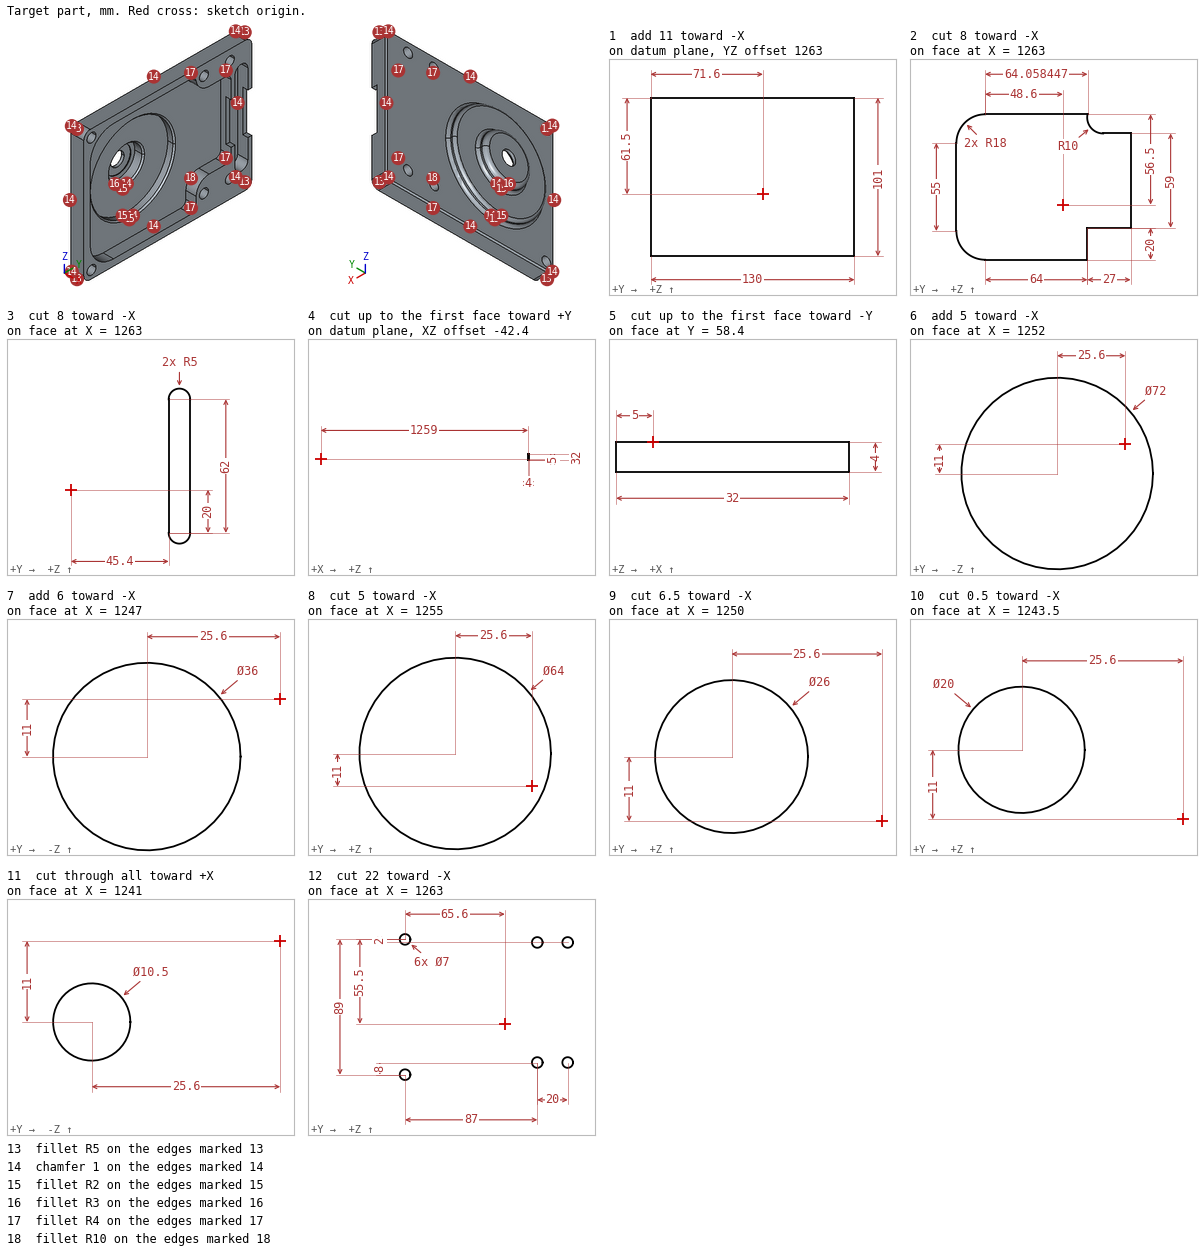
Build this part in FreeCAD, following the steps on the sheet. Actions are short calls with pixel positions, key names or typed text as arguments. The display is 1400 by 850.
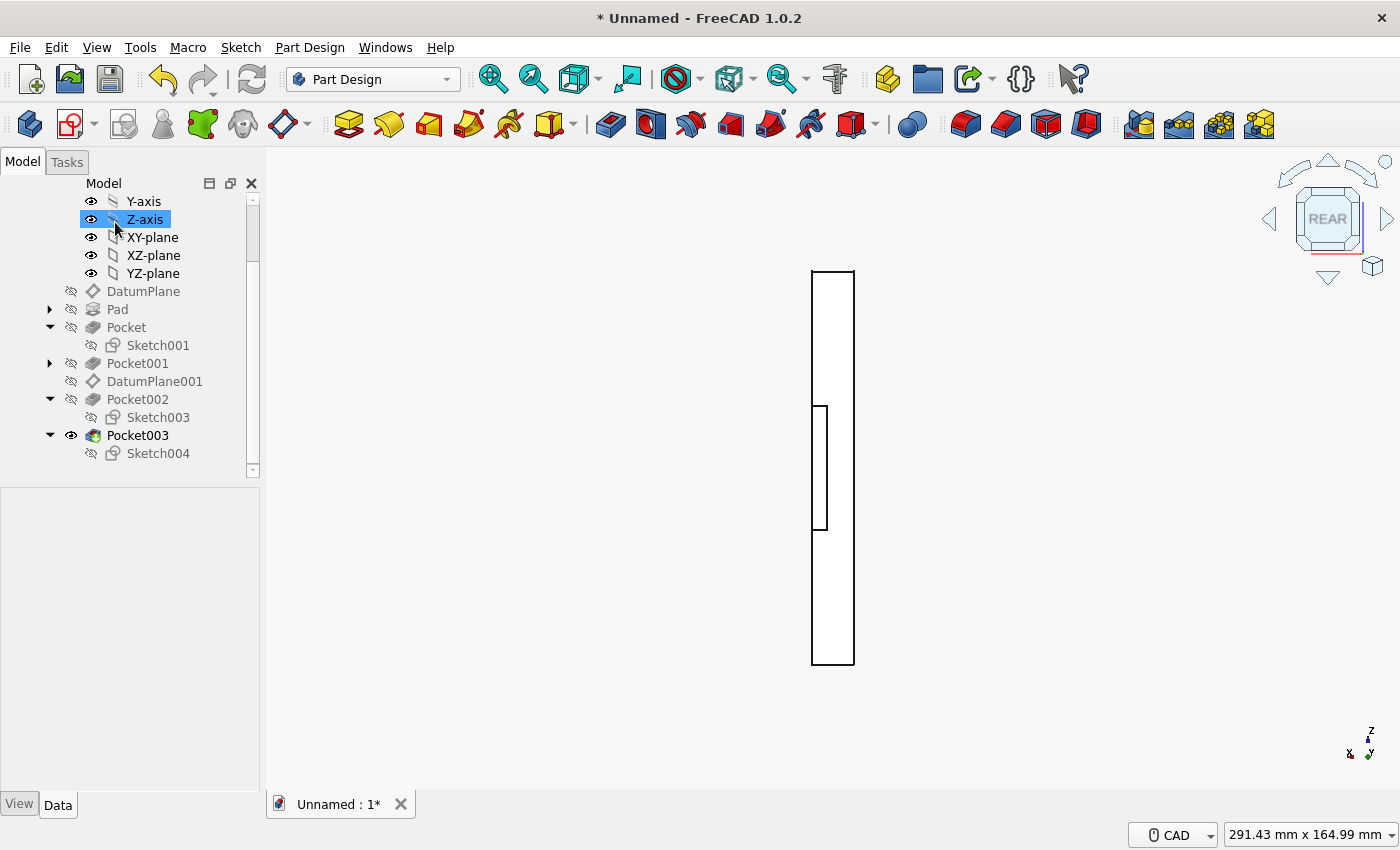
key(6)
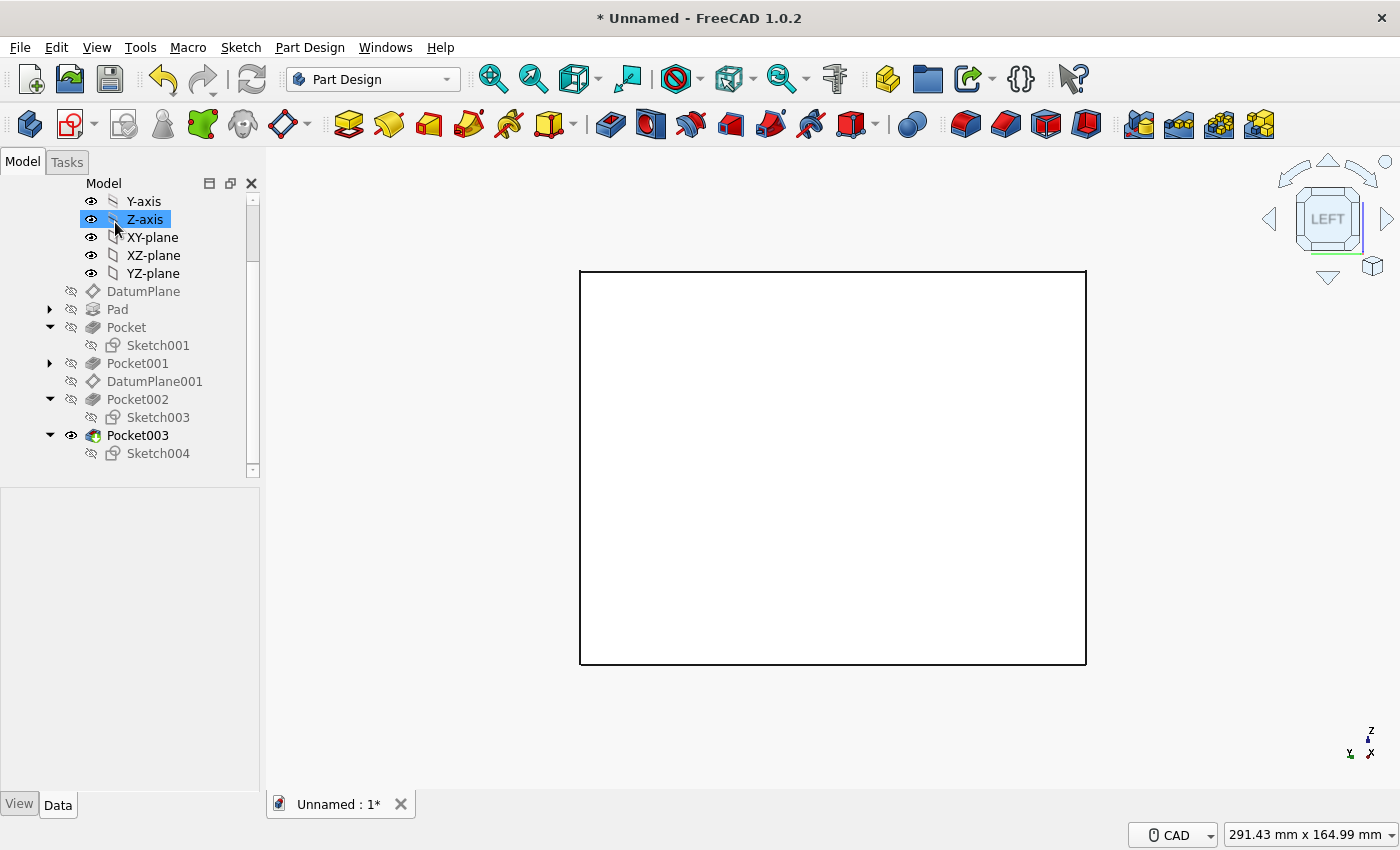
click(833, 467)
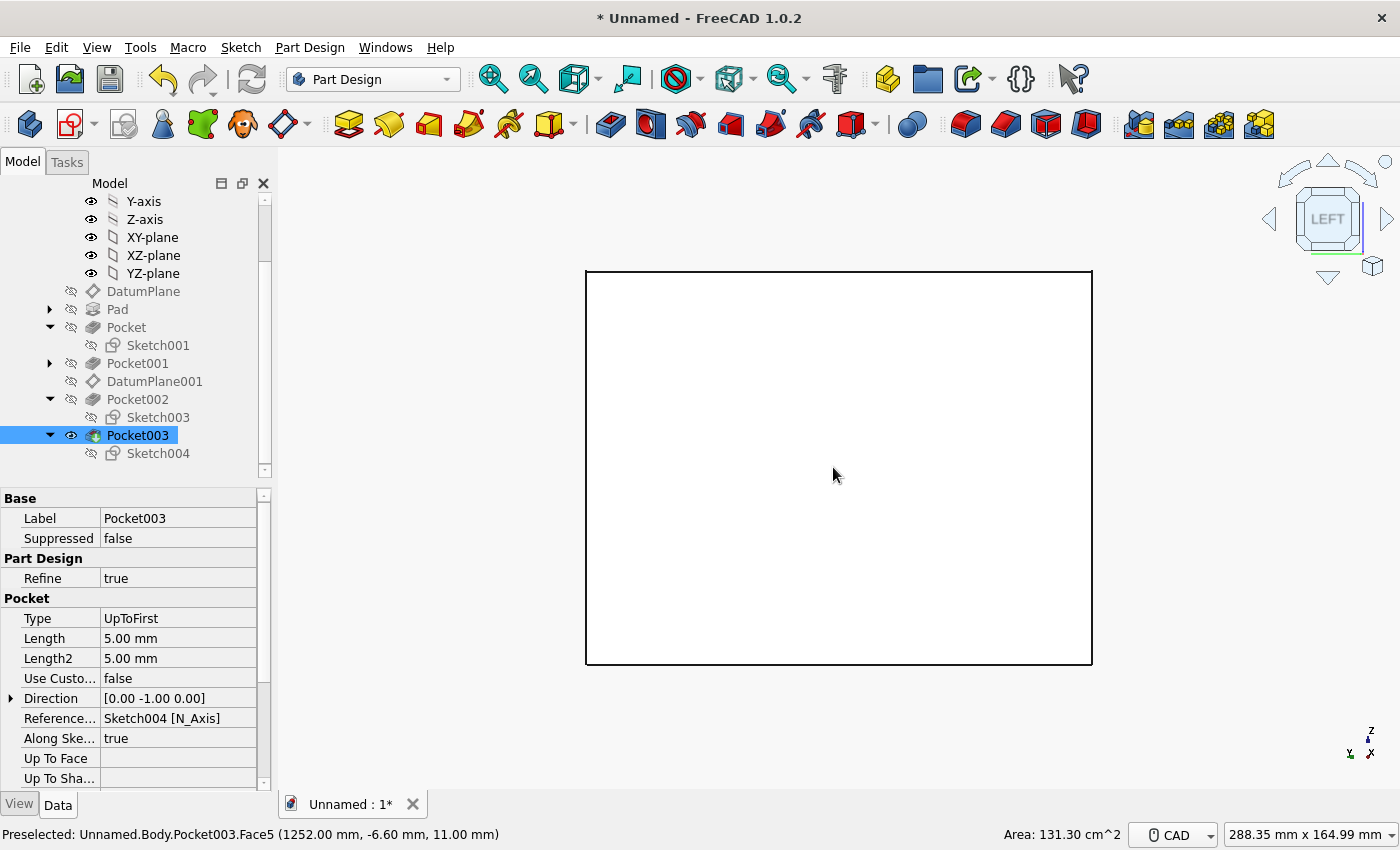
click(70, 124)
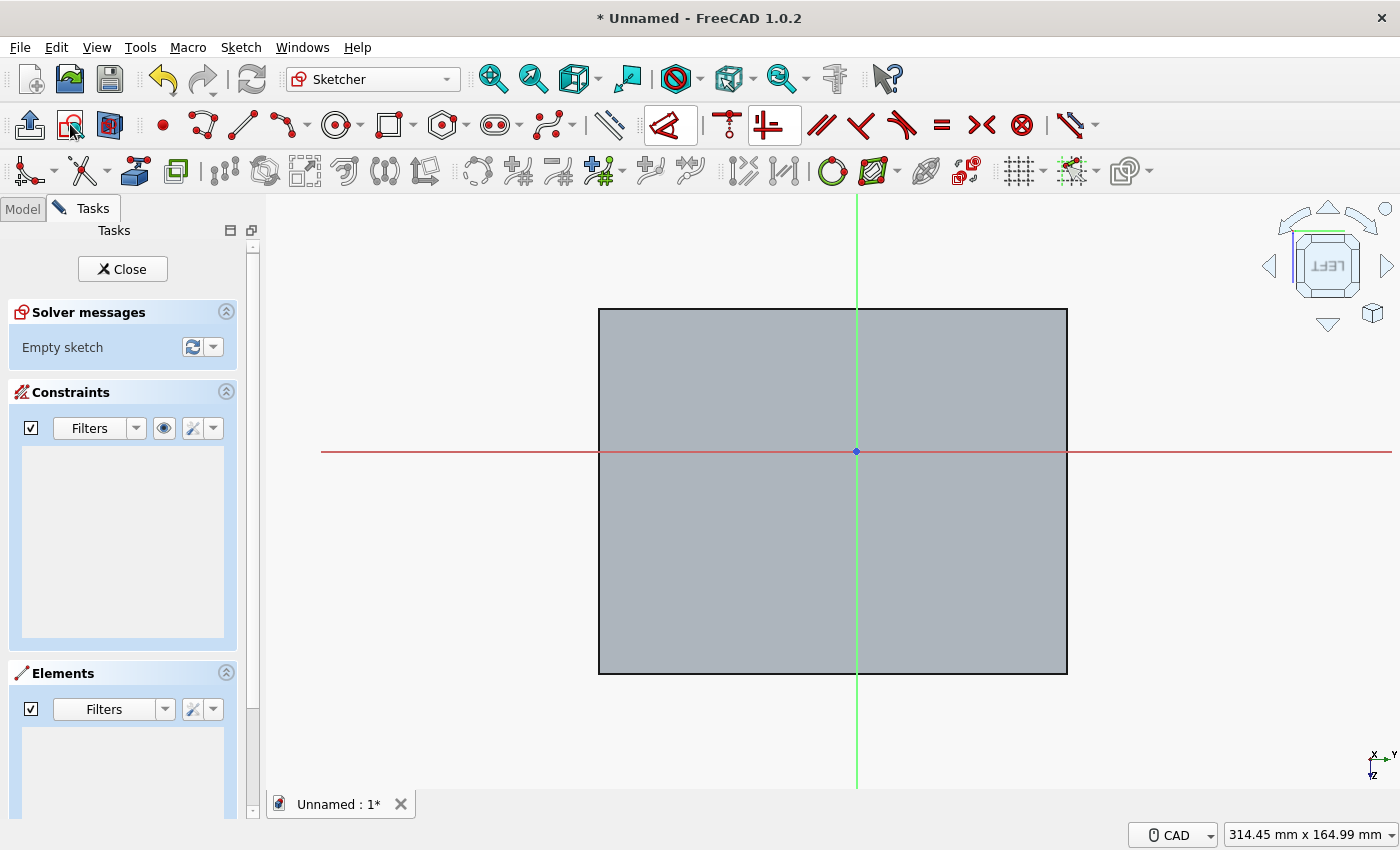
scroll(764, 491, up, 2)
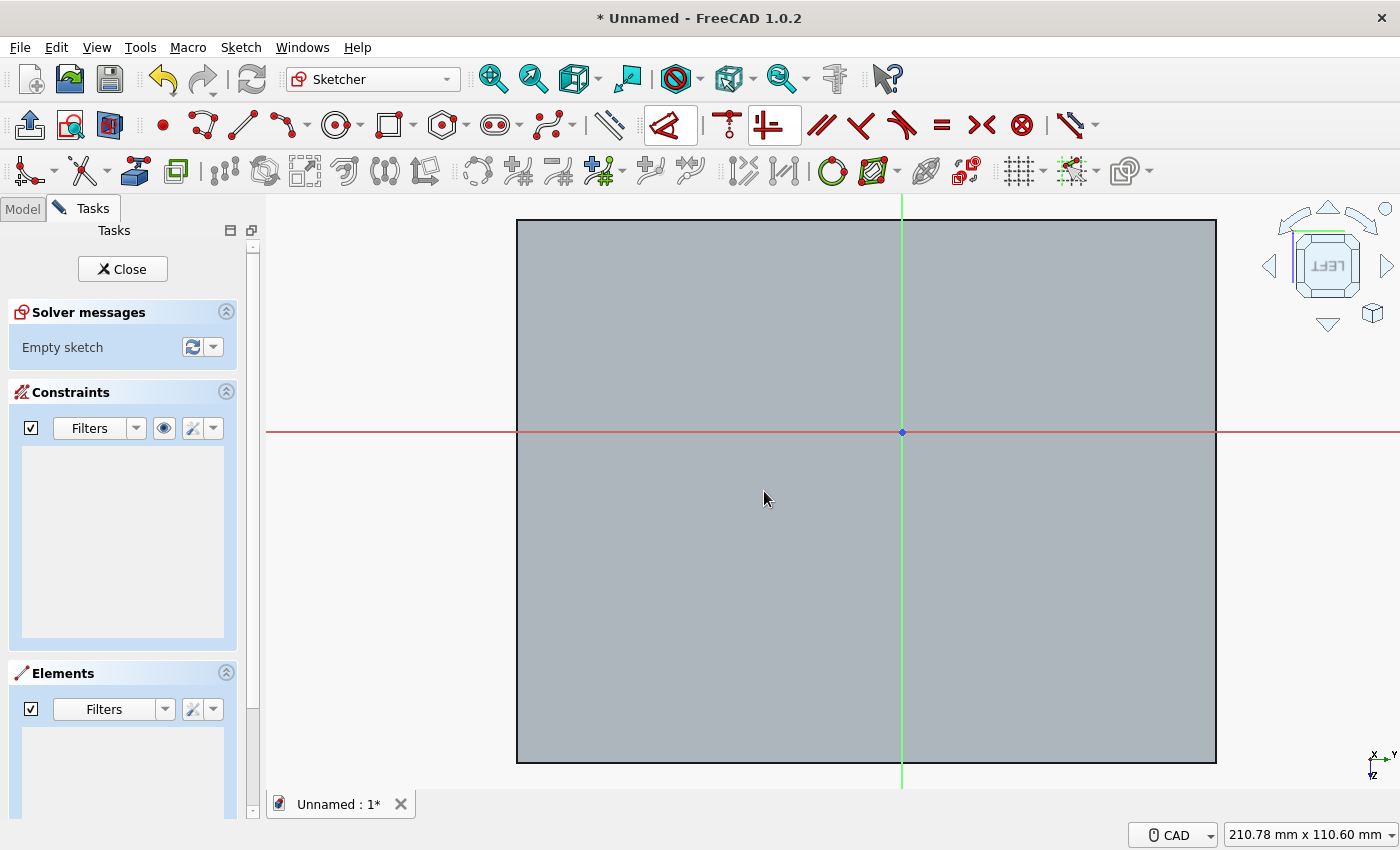
key(g)
key(c)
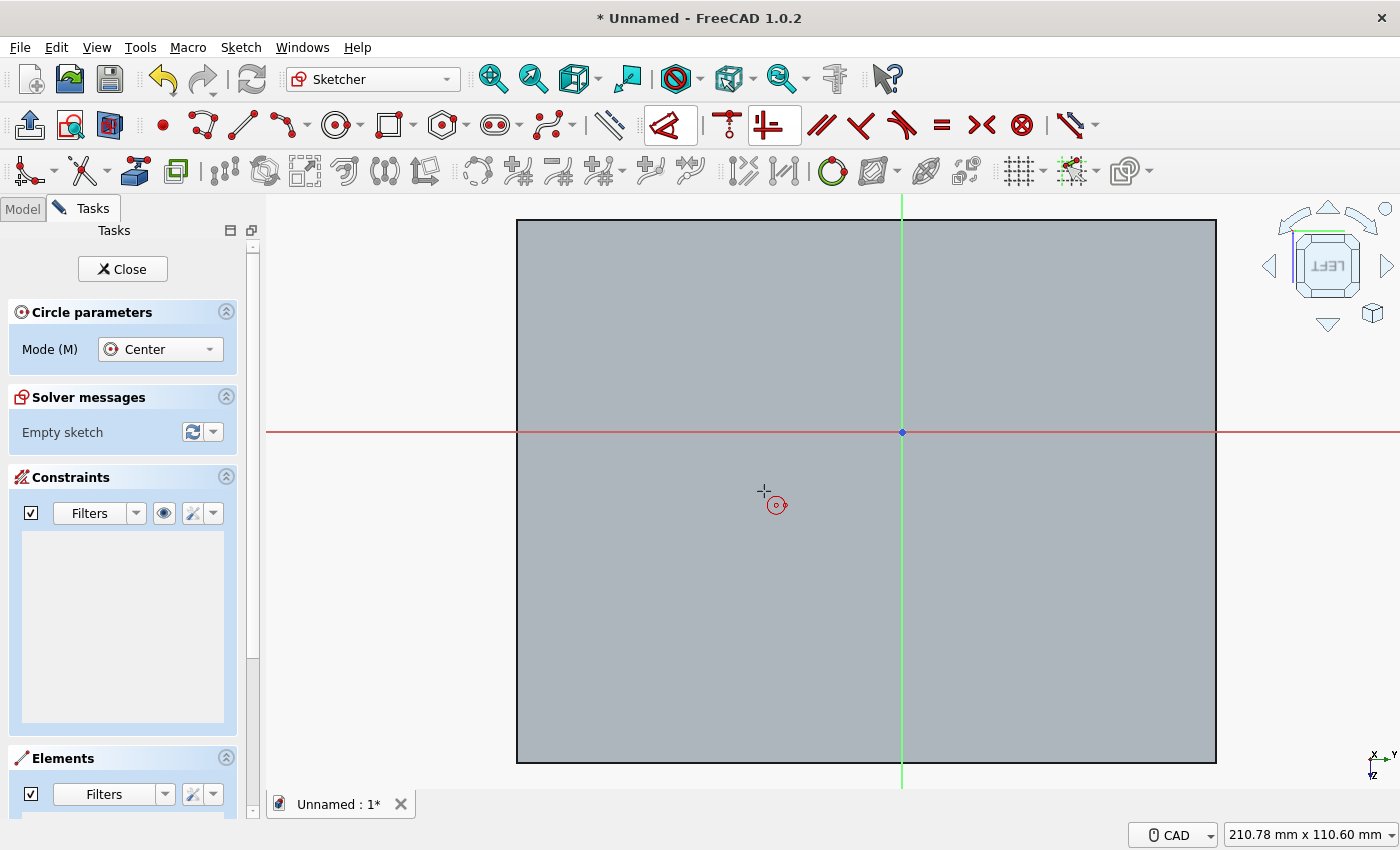
click(765, 491)
move(628, 355)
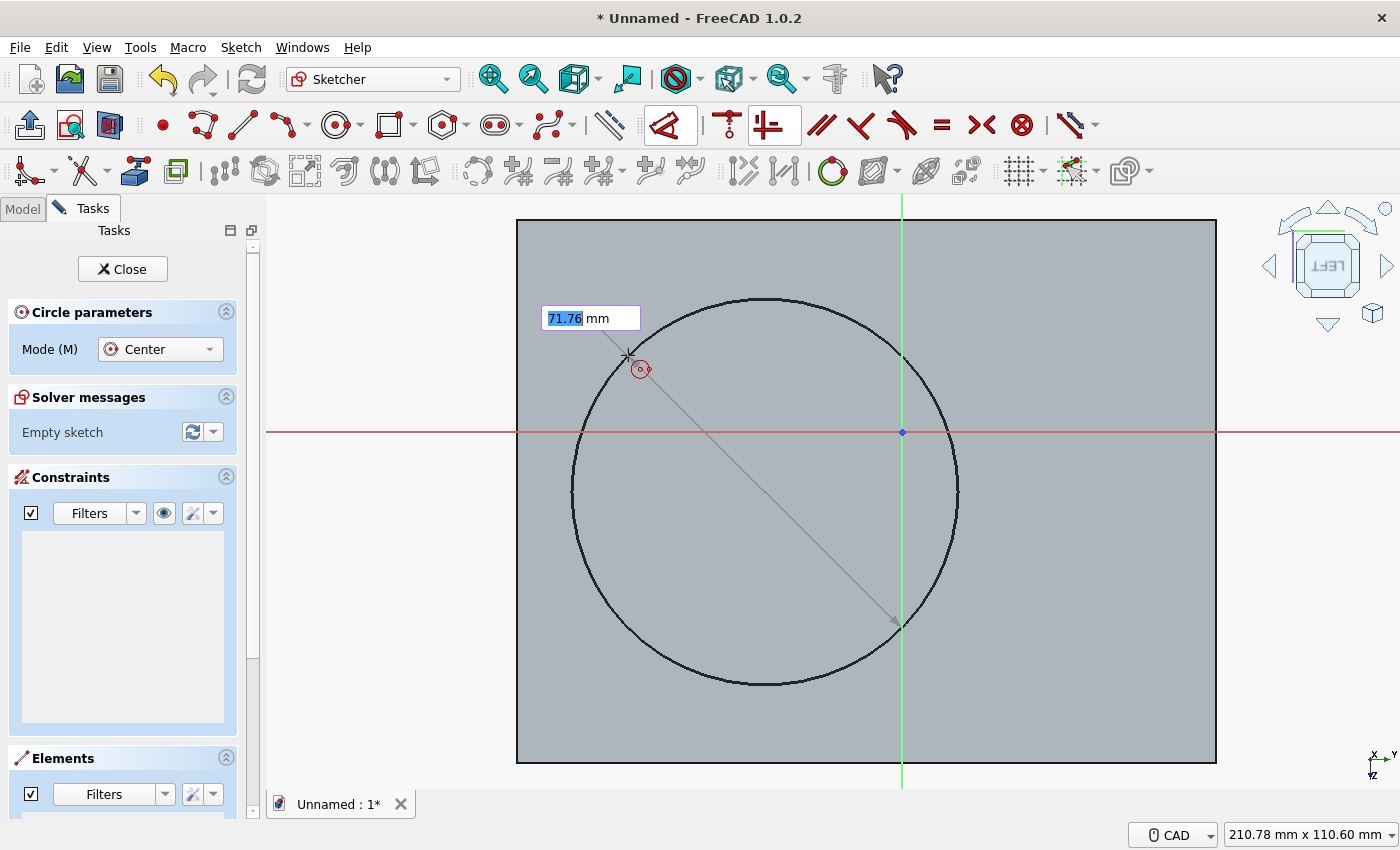
text(72)
key(Return)
key(Escape)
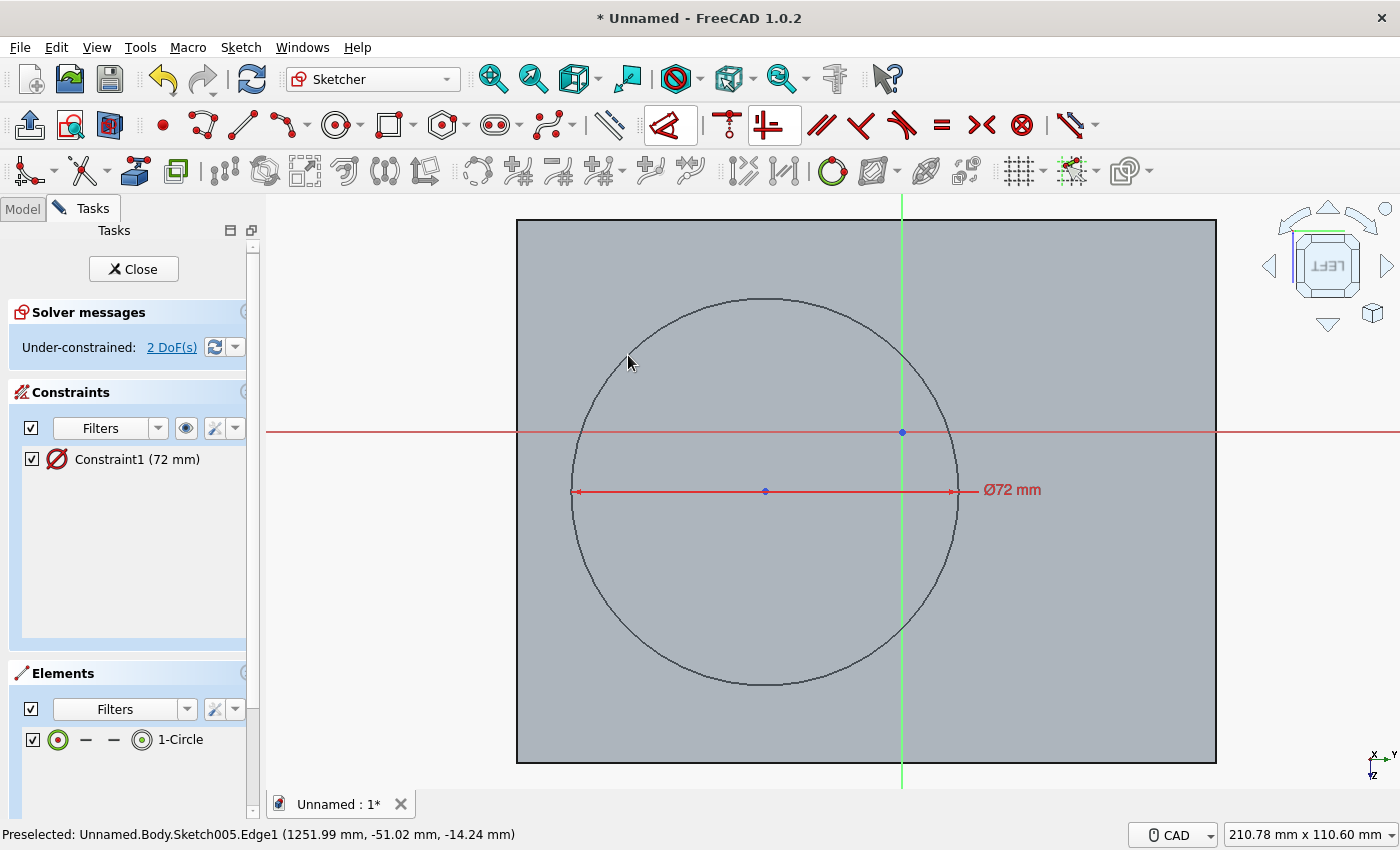
click(765, 492)